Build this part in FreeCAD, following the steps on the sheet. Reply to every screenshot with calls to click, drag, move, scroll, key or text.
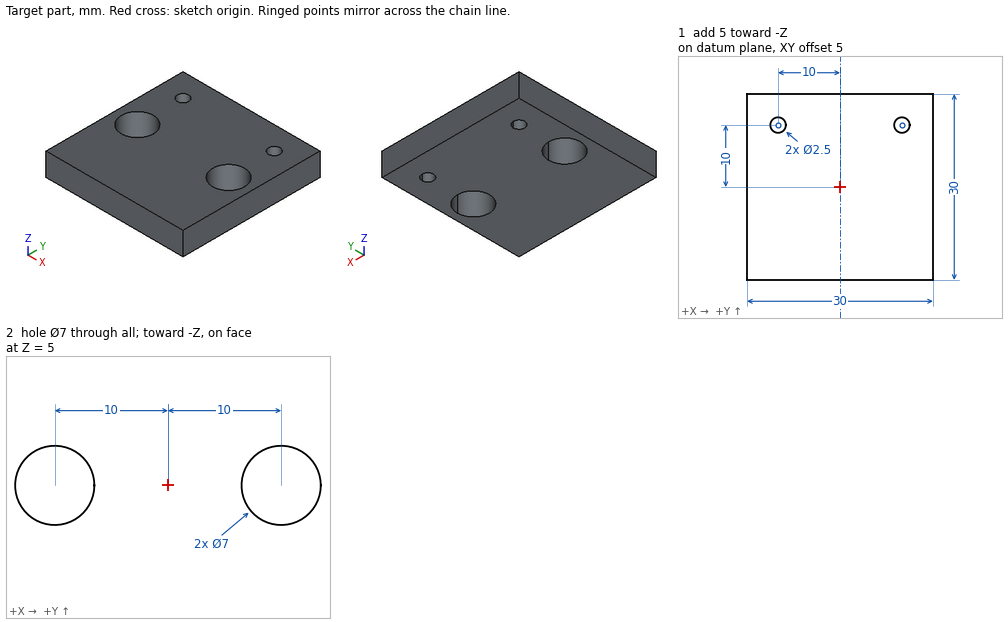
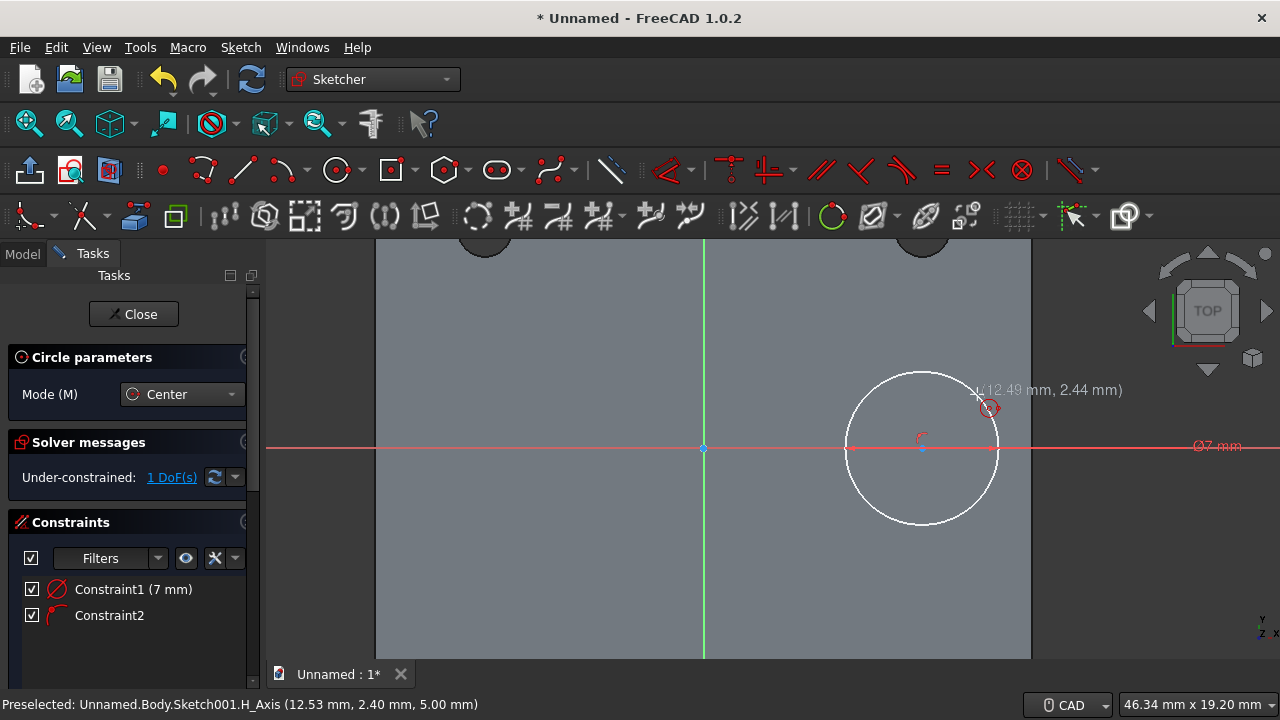
click(485, 448)
move(539, 394)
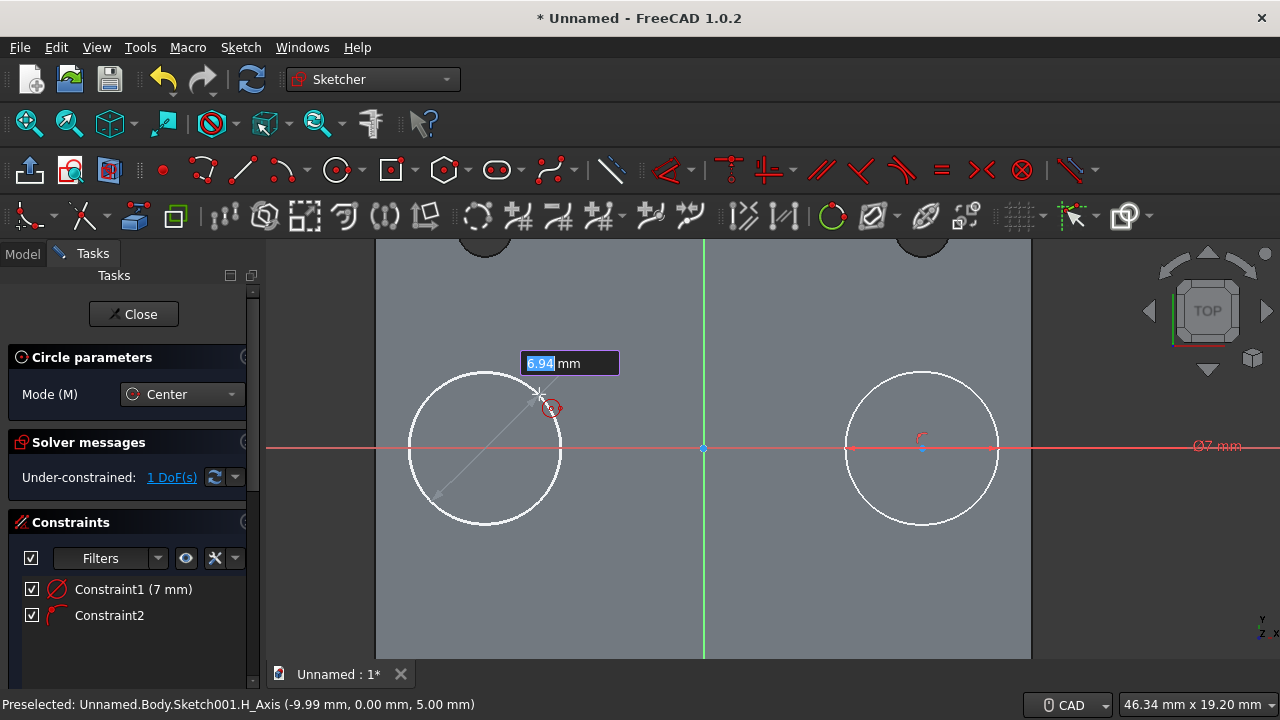
text(7)
key(Return)
key(Escape)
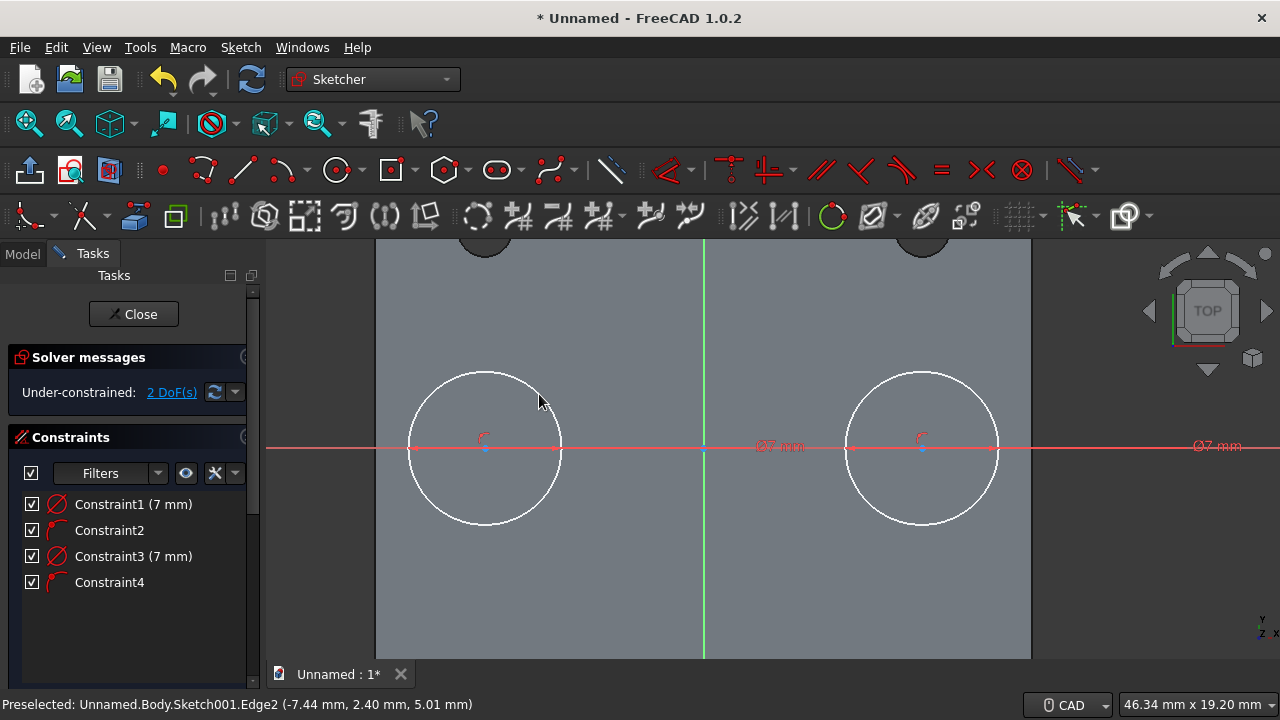
key(d)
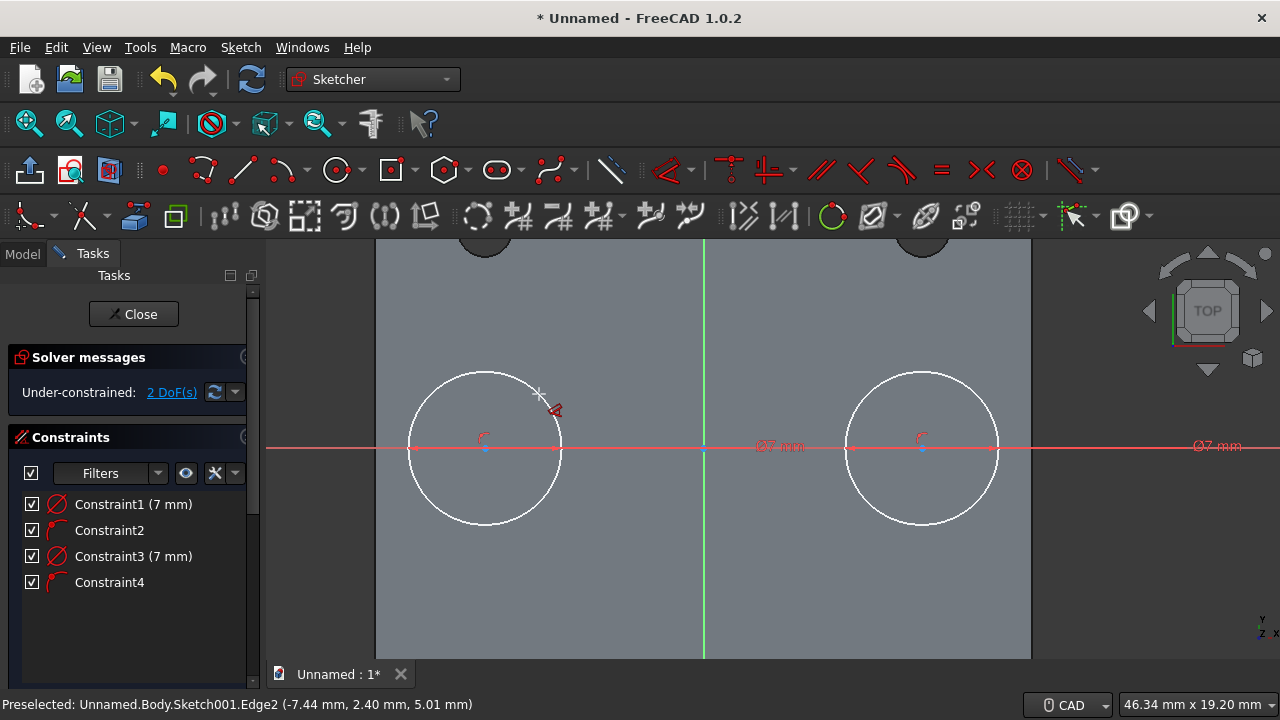
click(922, 448)
click(813, 482)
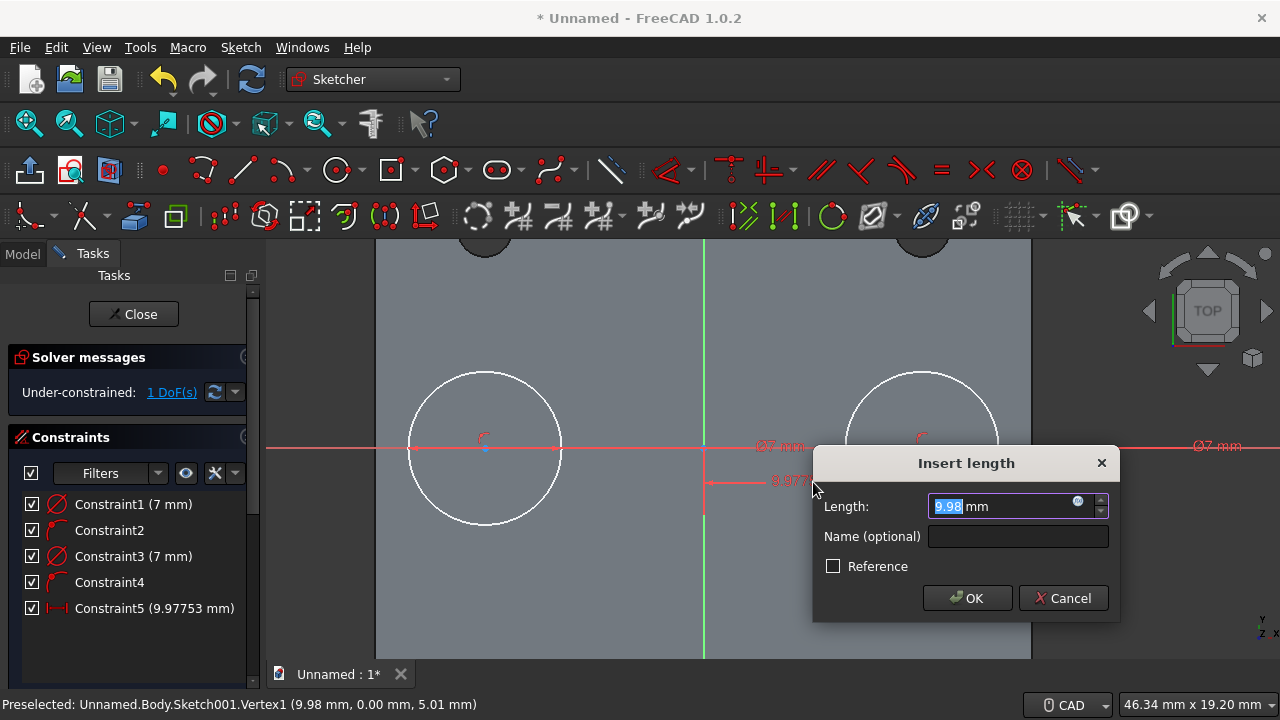
text(10)
key(Return)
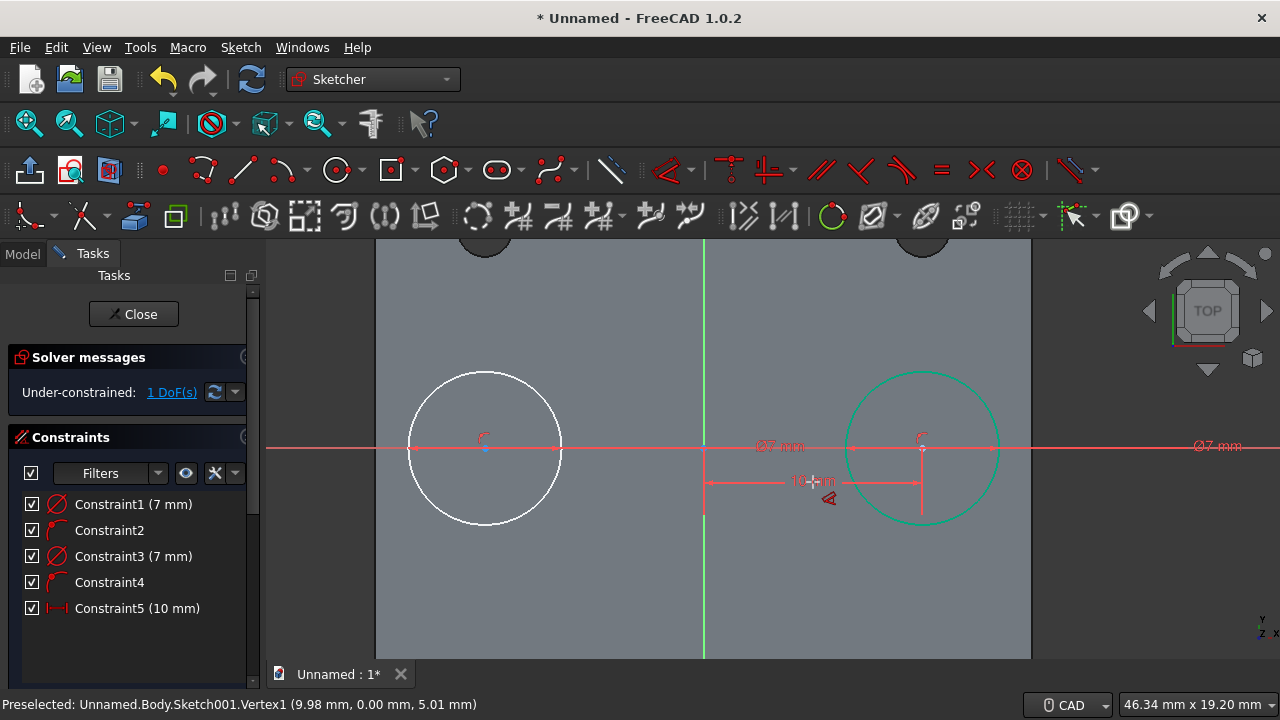
click(485, 448)
click(594, 482)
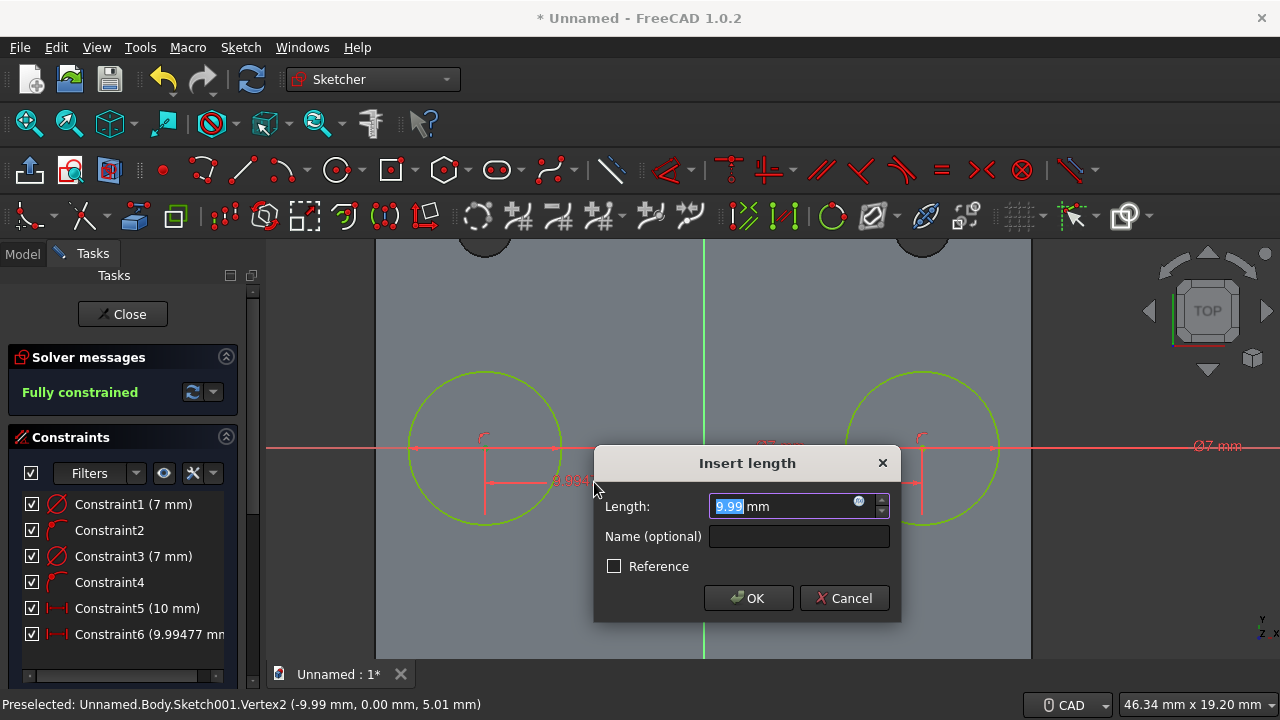
text(10)
key(Return)
key(Escape)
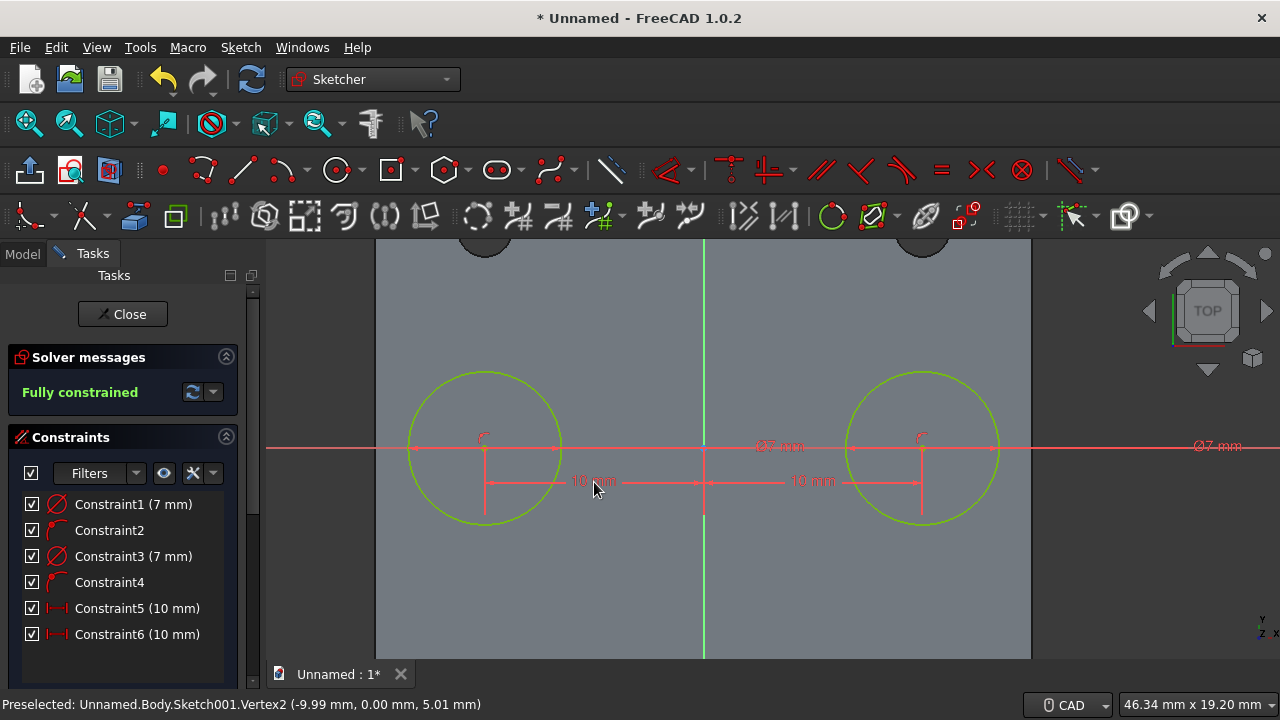
click(123, 314)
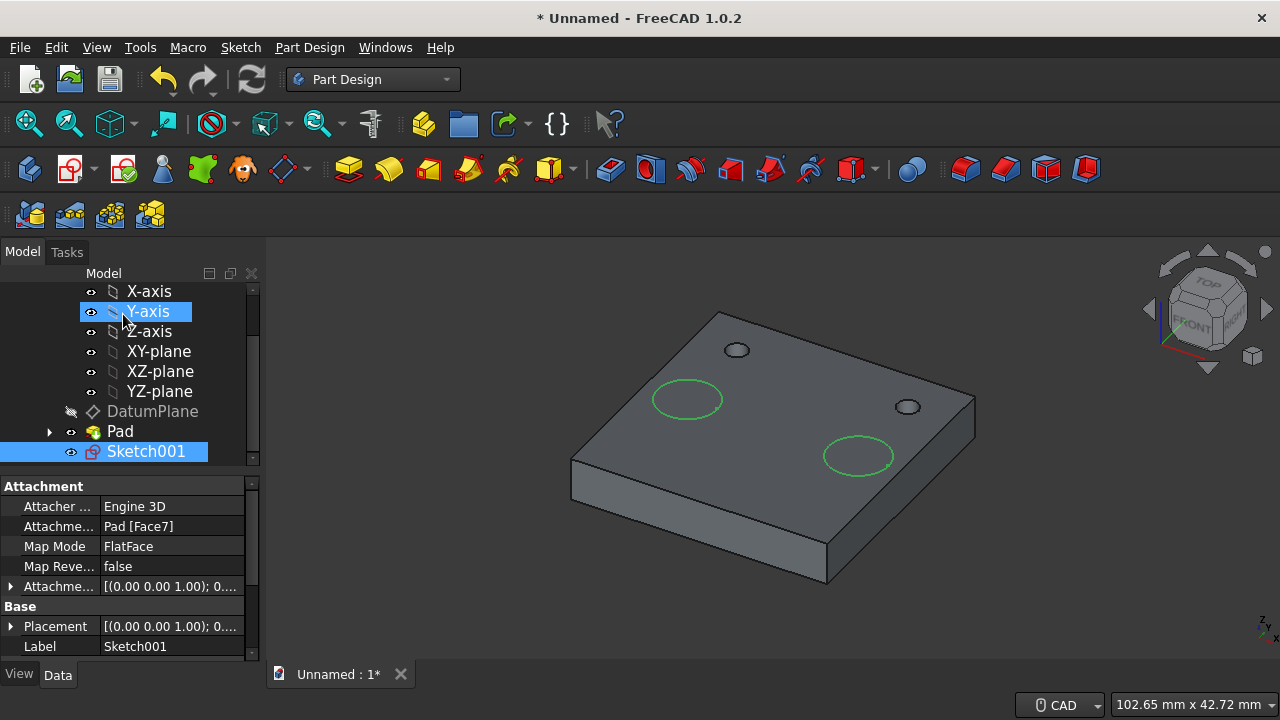
click(652, 170)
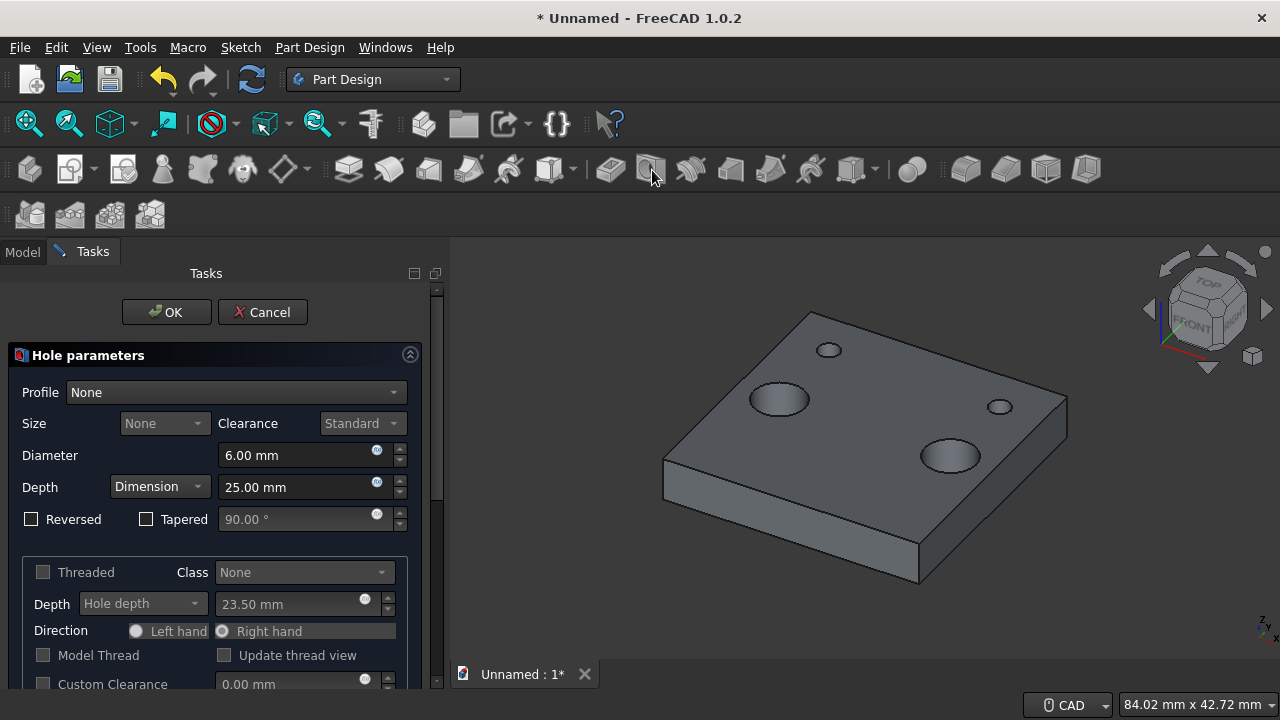
triple_click(305, 455)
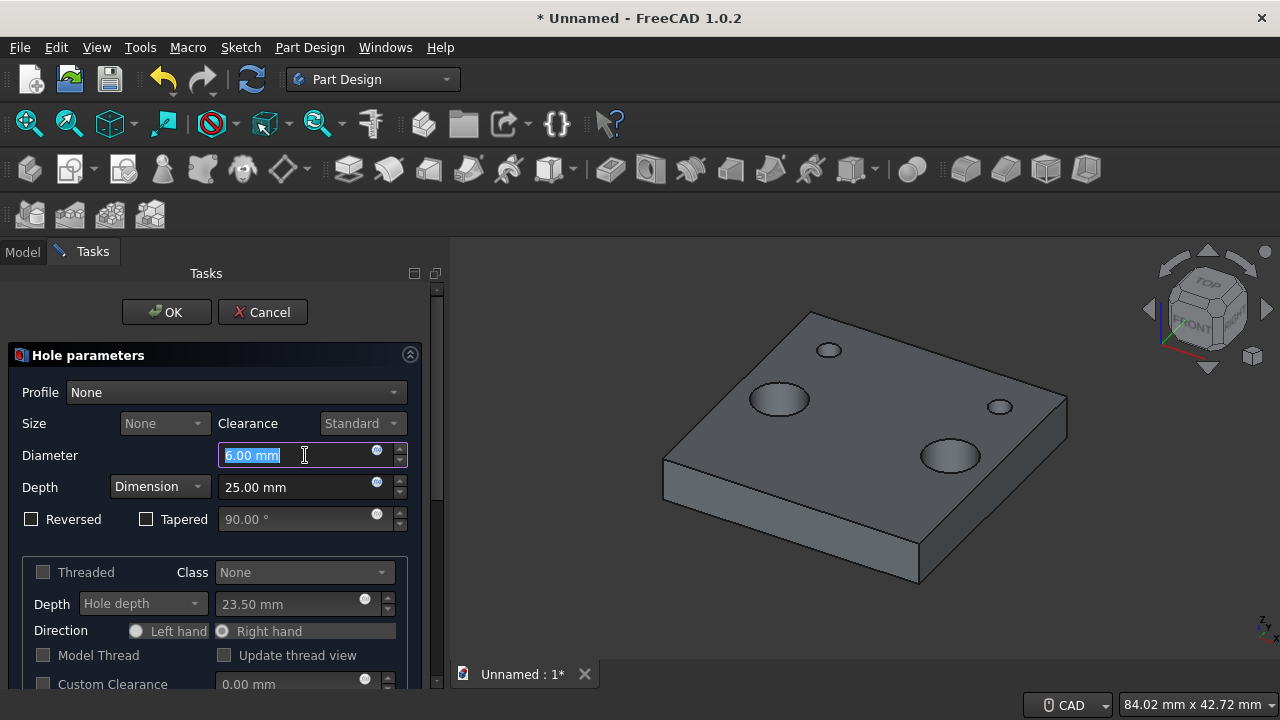
text(7)
key(Tab)